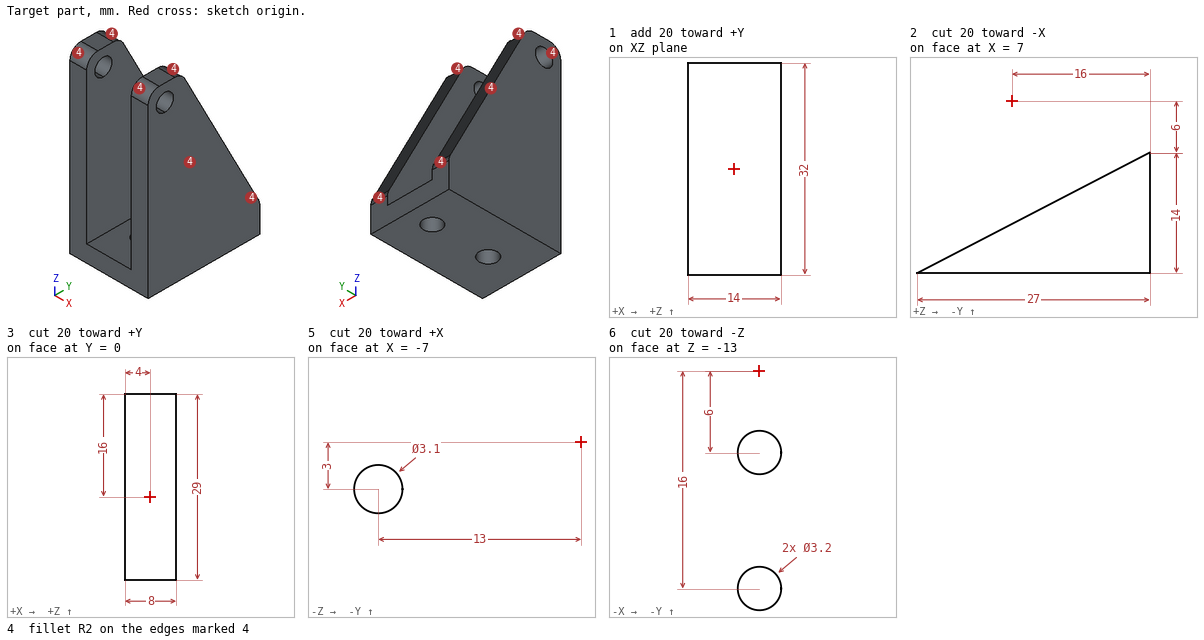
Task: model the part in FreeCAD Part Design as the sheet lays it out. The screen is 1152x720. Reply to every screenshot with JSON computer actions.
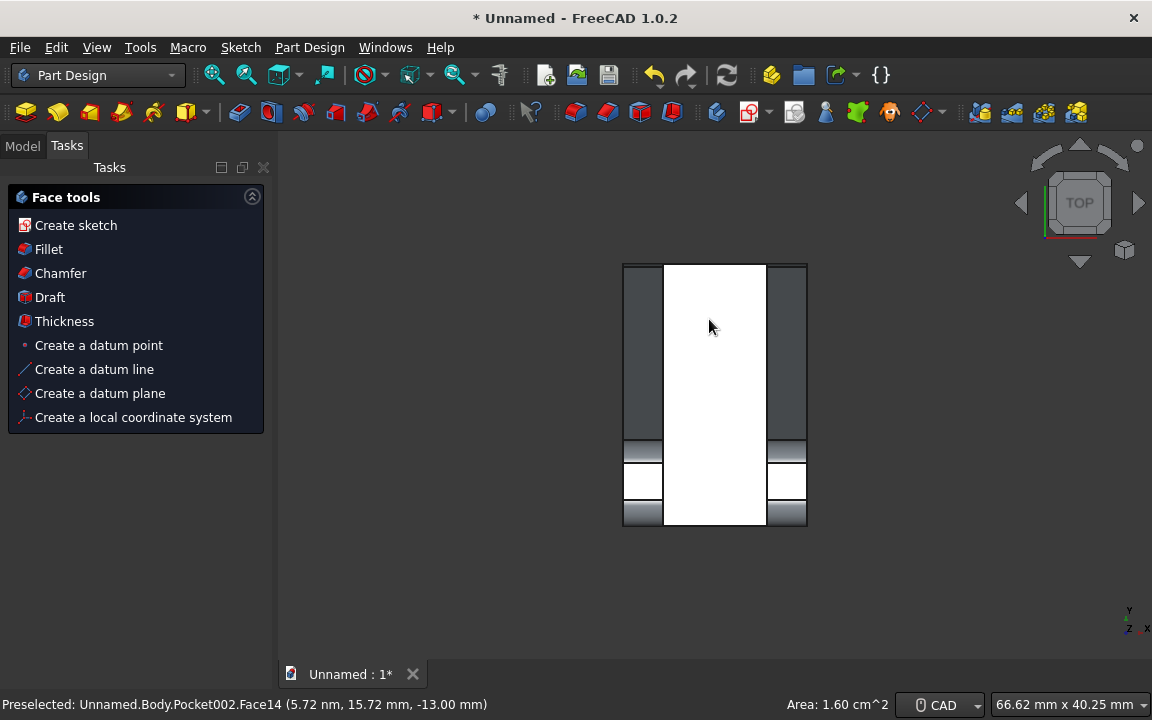
{"action": "left_click", "coordinate": [750, 112]}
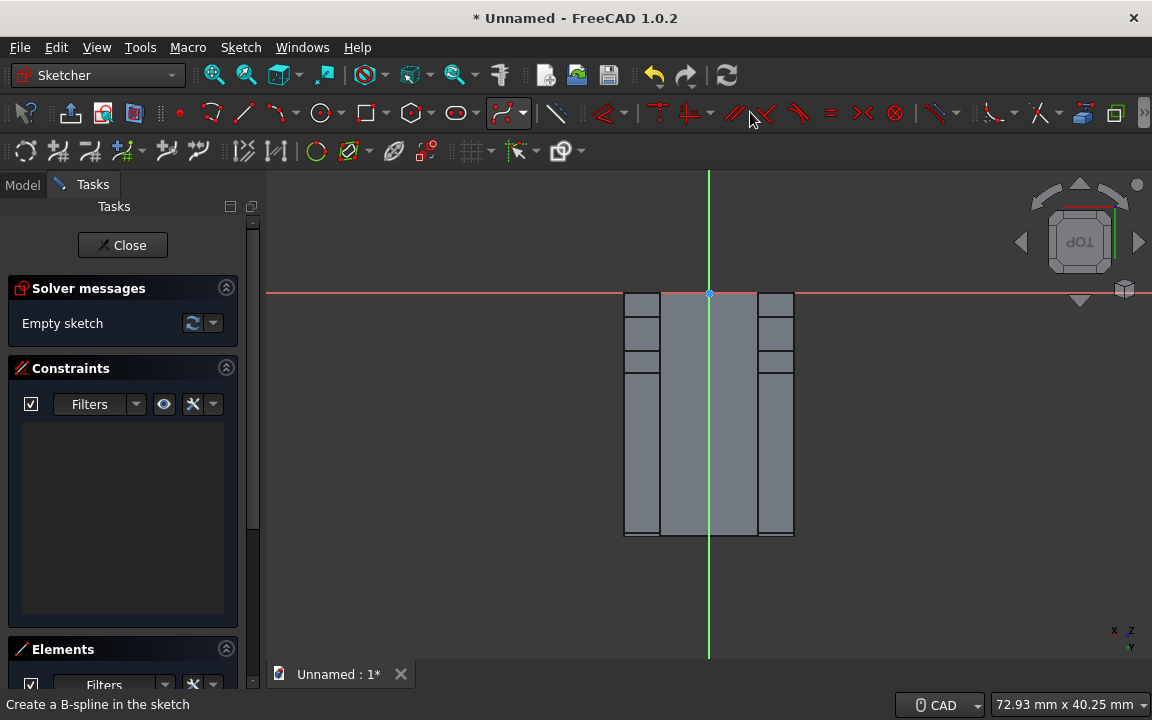
{"action": "scroll", "coordinate": [848, 370], "scroll_direction": "up", "scroll_amount": 2}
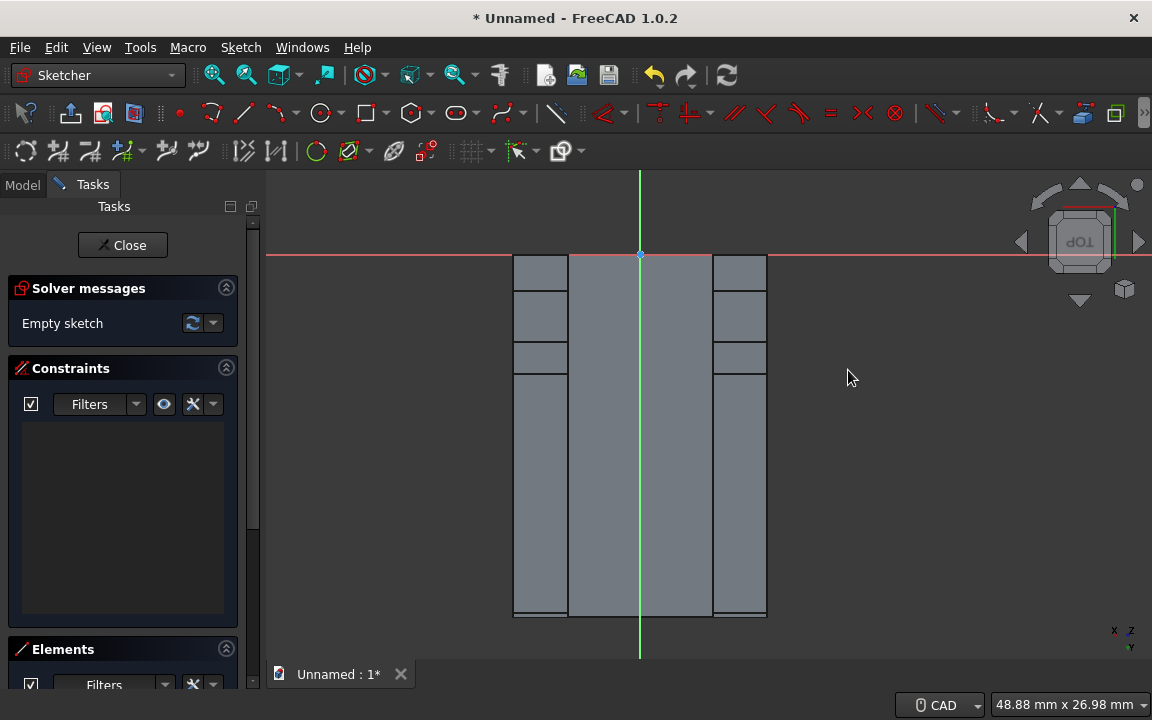
{"action": "left_click", "coordinate": [322, 114]}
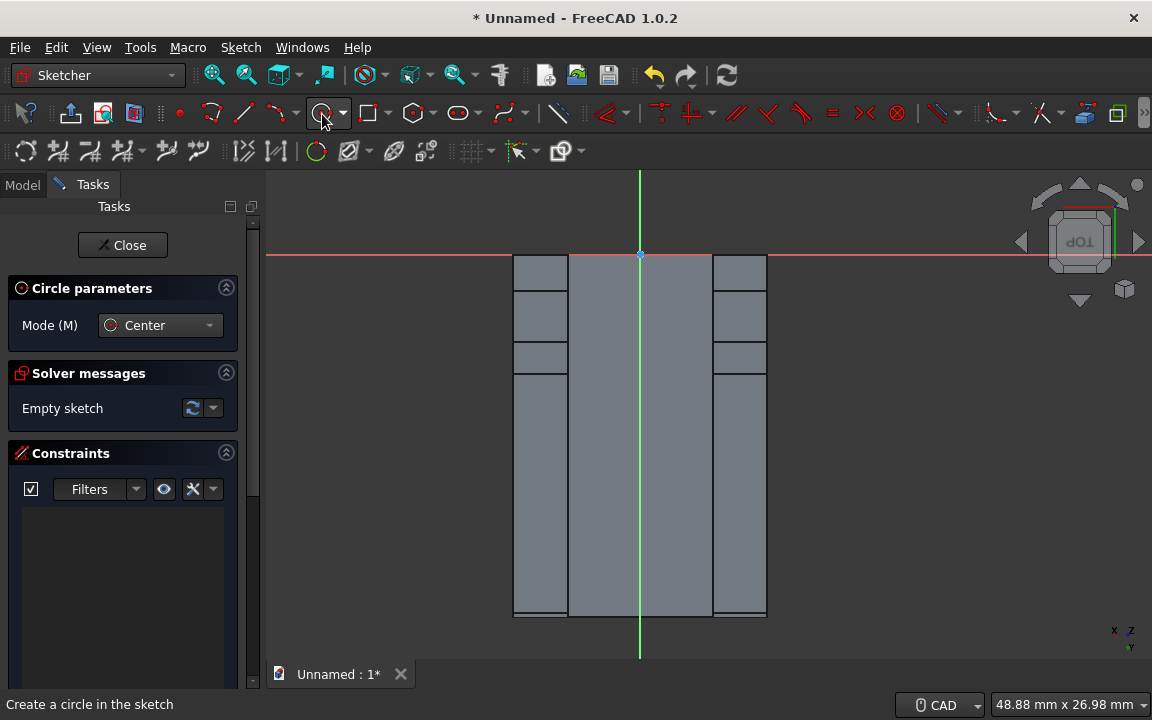
{"action": "left_click", "coordinate": [640, 545]}
{"action": "mouse_move", "coordinate": [661, 524]}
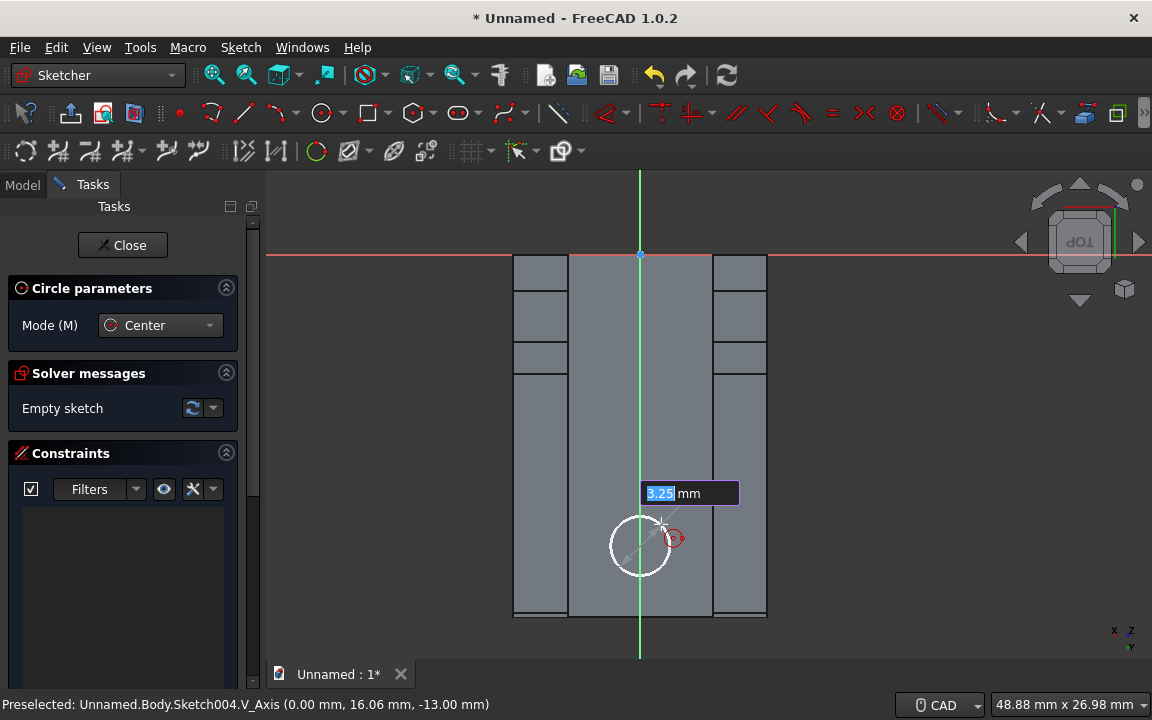
{"action": "type", "text": "3.2"}
{"action": "key", "text": "Return"}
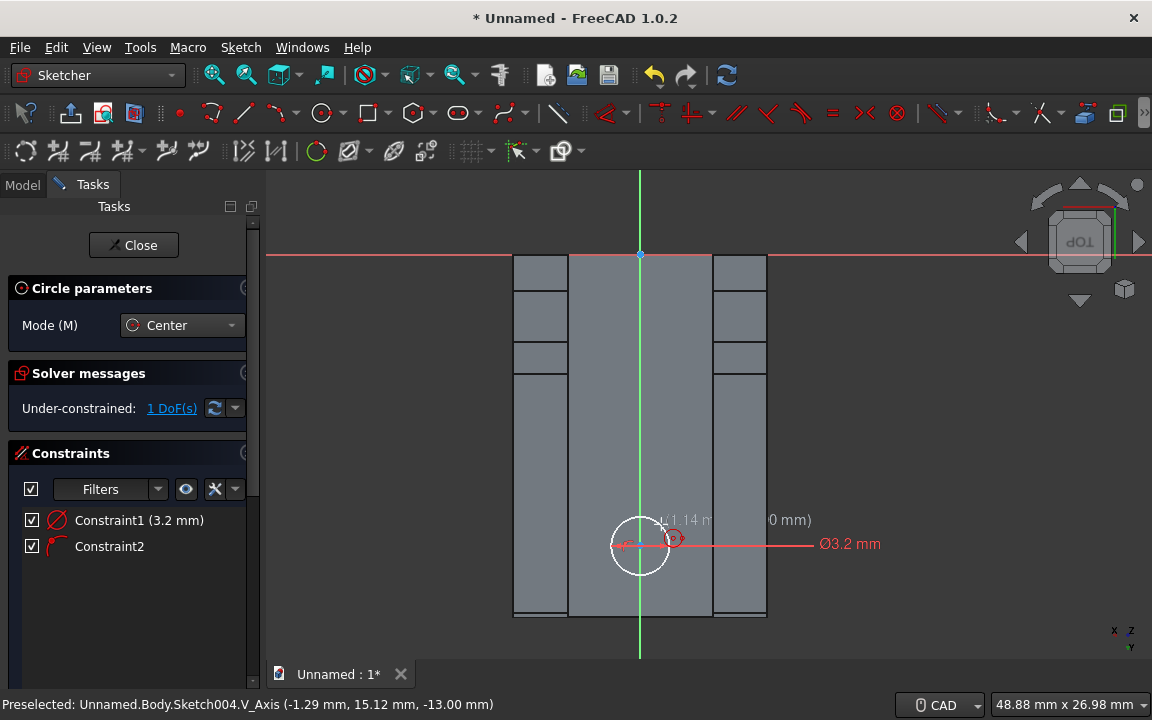
{"action": "left_click", "coordinate": [640, 364]}
{"action": "mouse_move", "coordinate": [661, 343]}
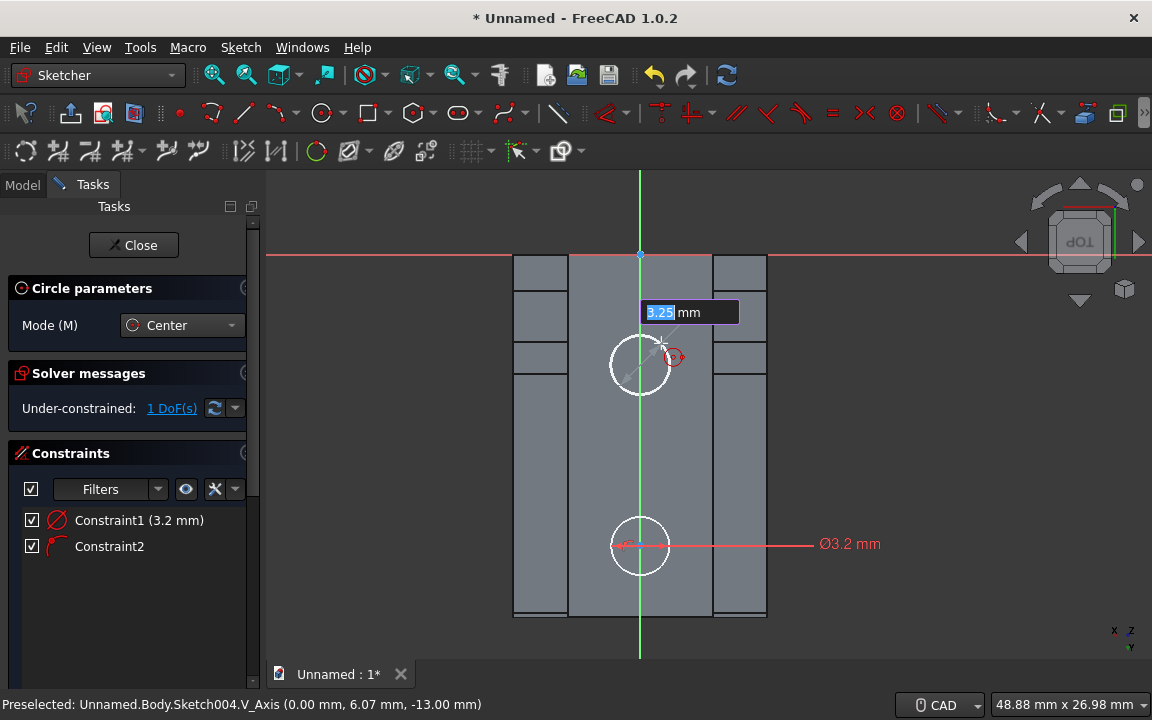
{"action": "type", "text": "3.2"}
{"action": "key", "text": "Return"}
{"action": "key", "text": "Escape"}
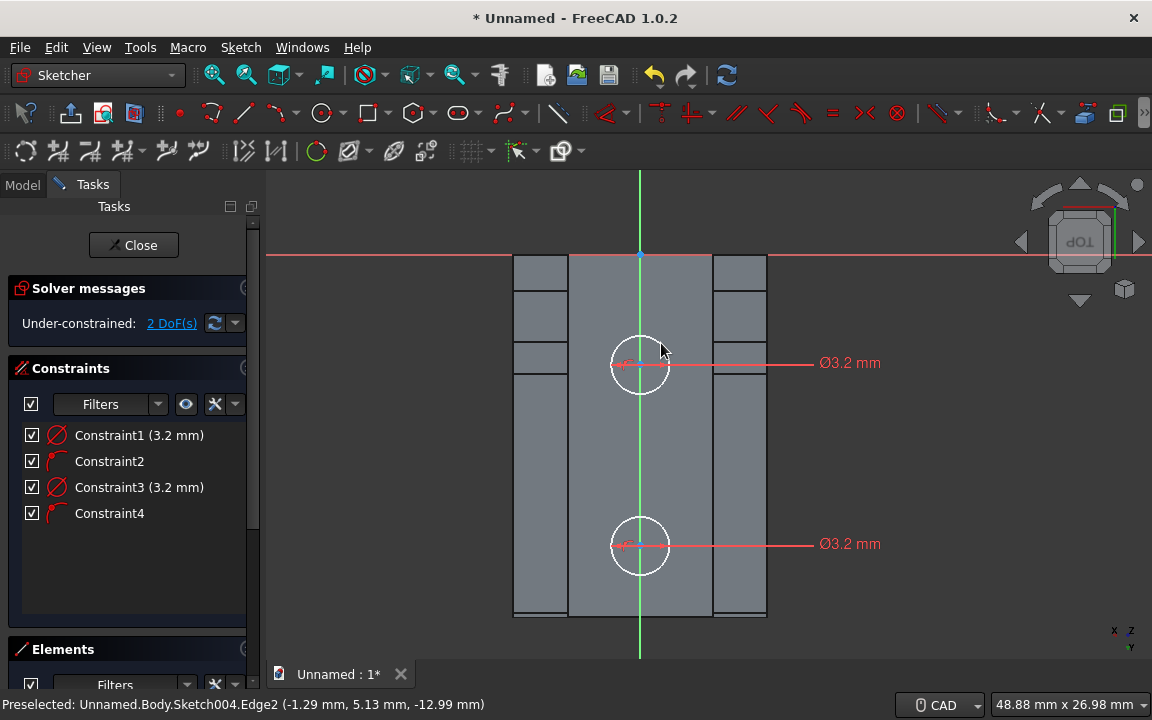
{"action": "left_click", "coordinate": [606, 114]}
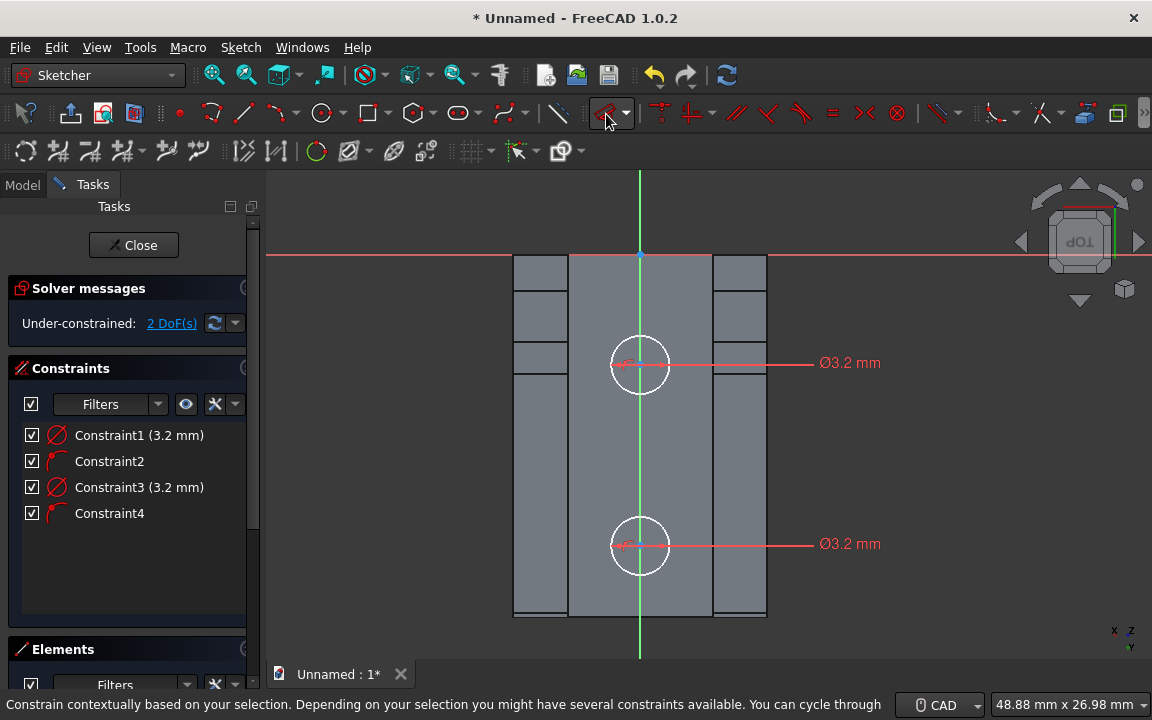
{"action": "left_click", "coordinate": [640, 365]}
{"action": "left_click", "coordinate": [674, 310]}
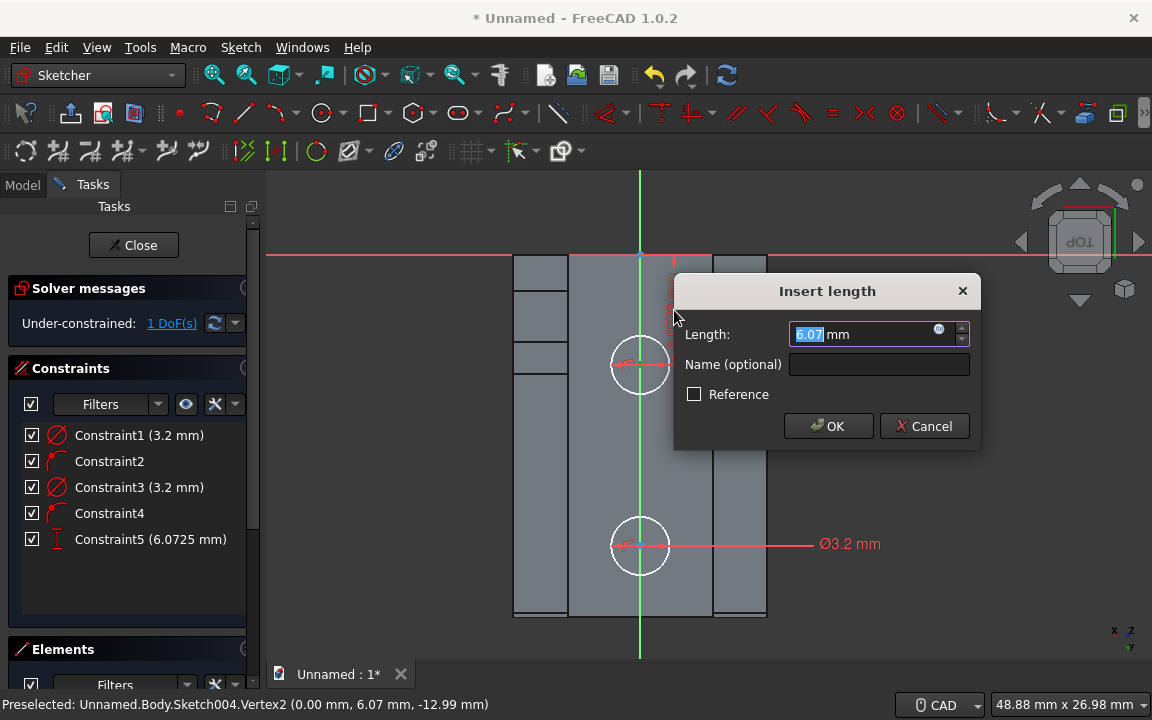
{"action": "type", "text": "6"}
{"action": "key", "text": "Return"}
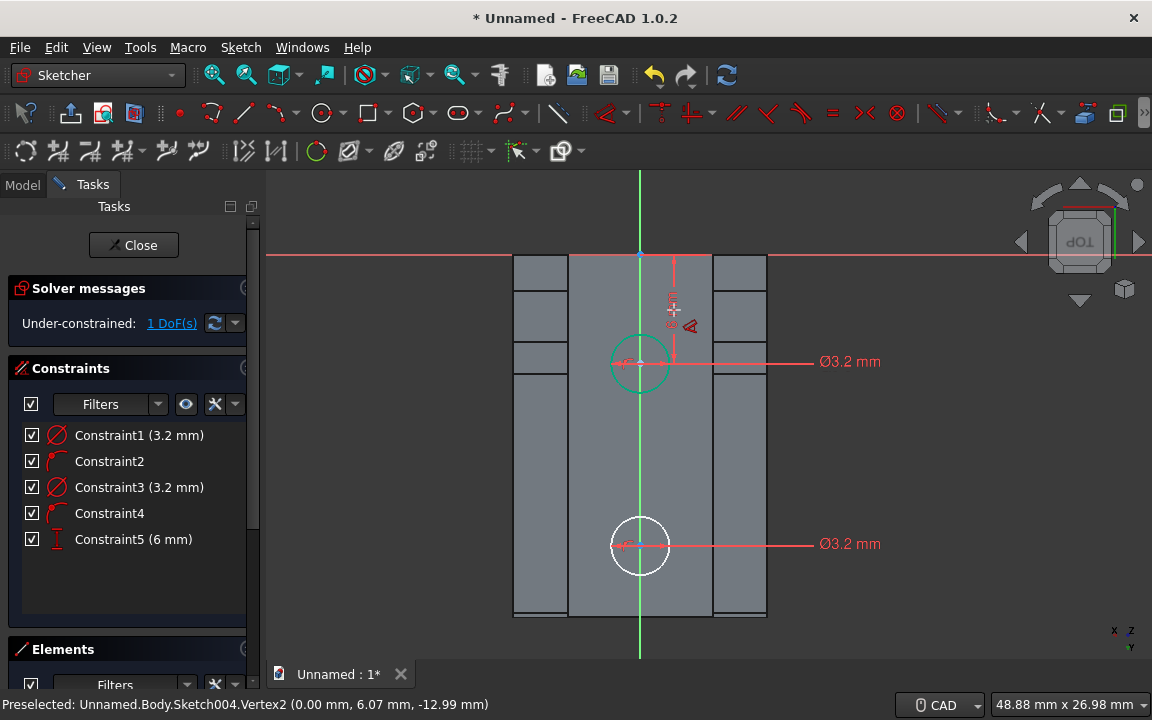
{"action": "left_click", "coordinate": [640, 546]}
{"action": "left_click", "coordinate": [674, 400]}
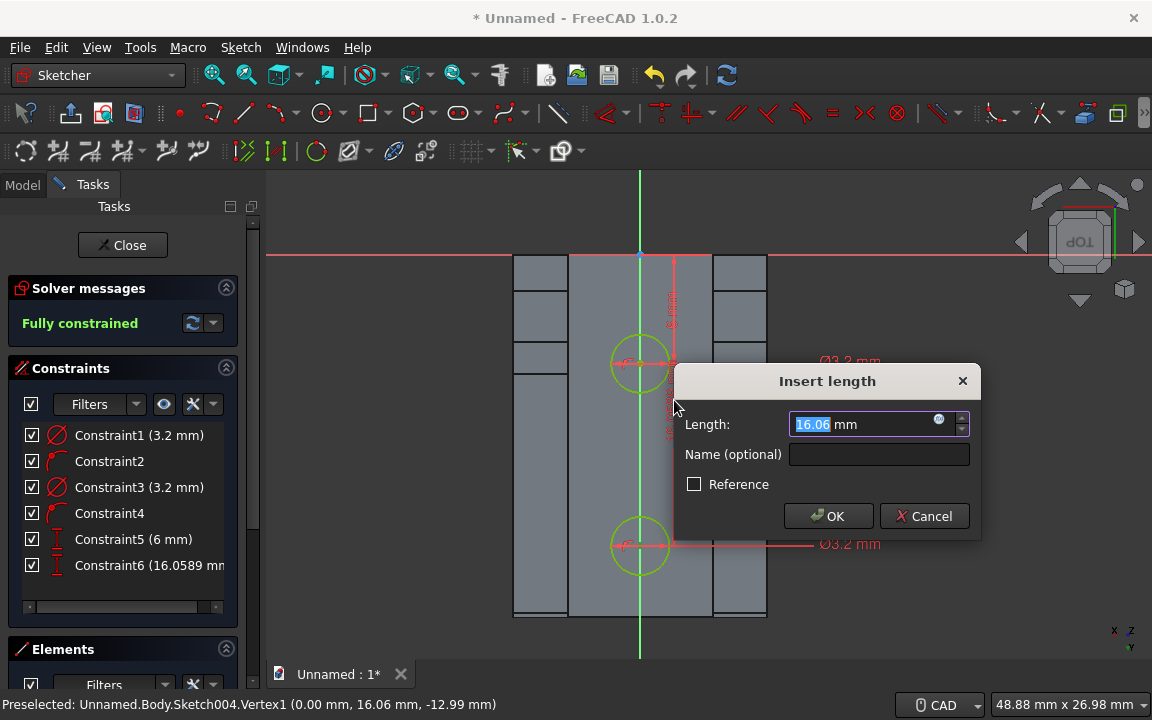
{"action": "type", "text": "16"}
{"action": "key", "text": "Return"}
{"action": "key", "text": "Escape"}